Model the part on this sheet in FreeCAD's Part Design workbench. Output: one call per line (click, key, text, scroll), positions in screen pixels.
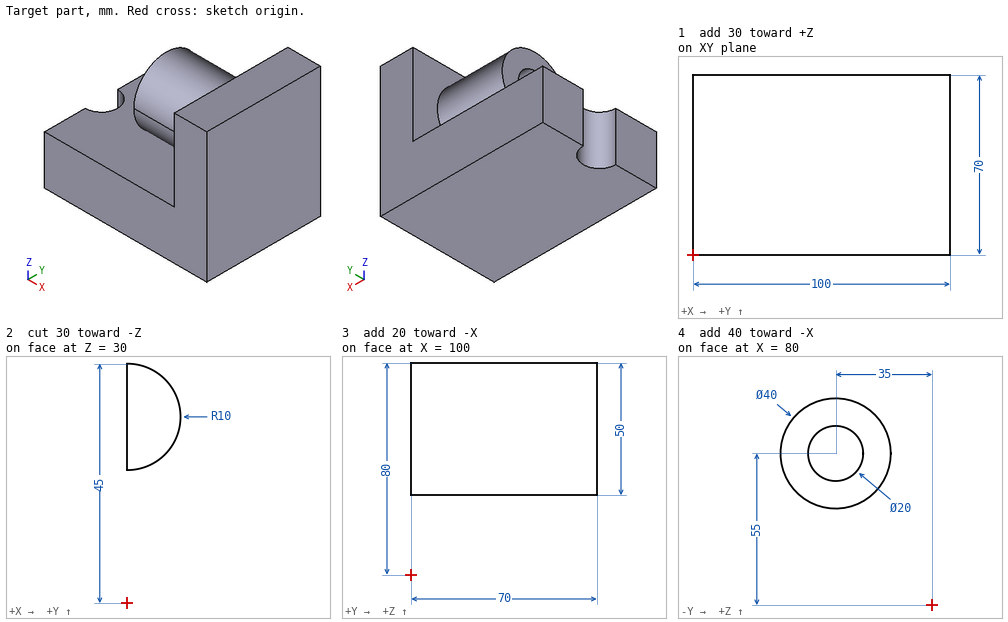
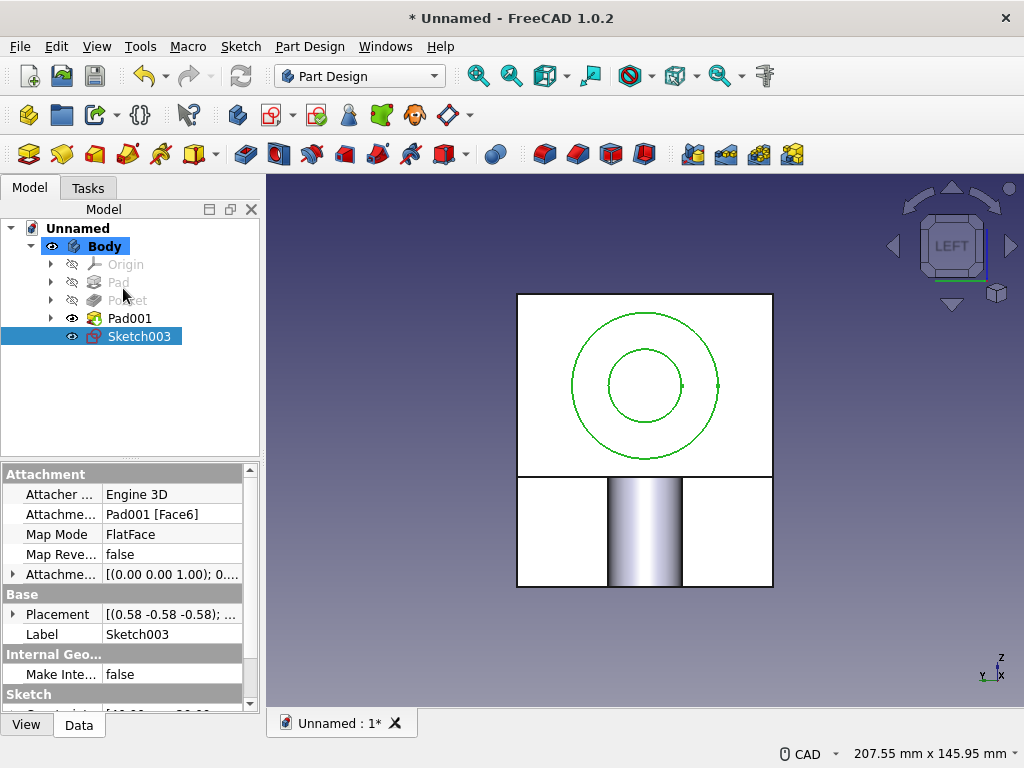
click(29, 154)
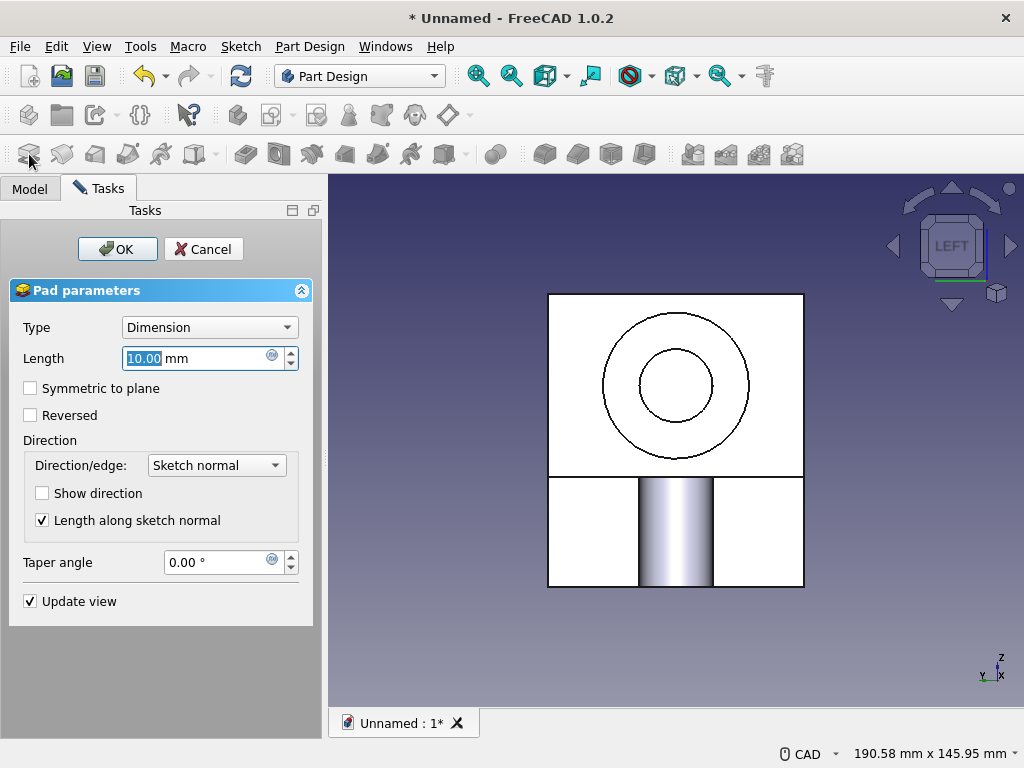
text(40)
key(Tab)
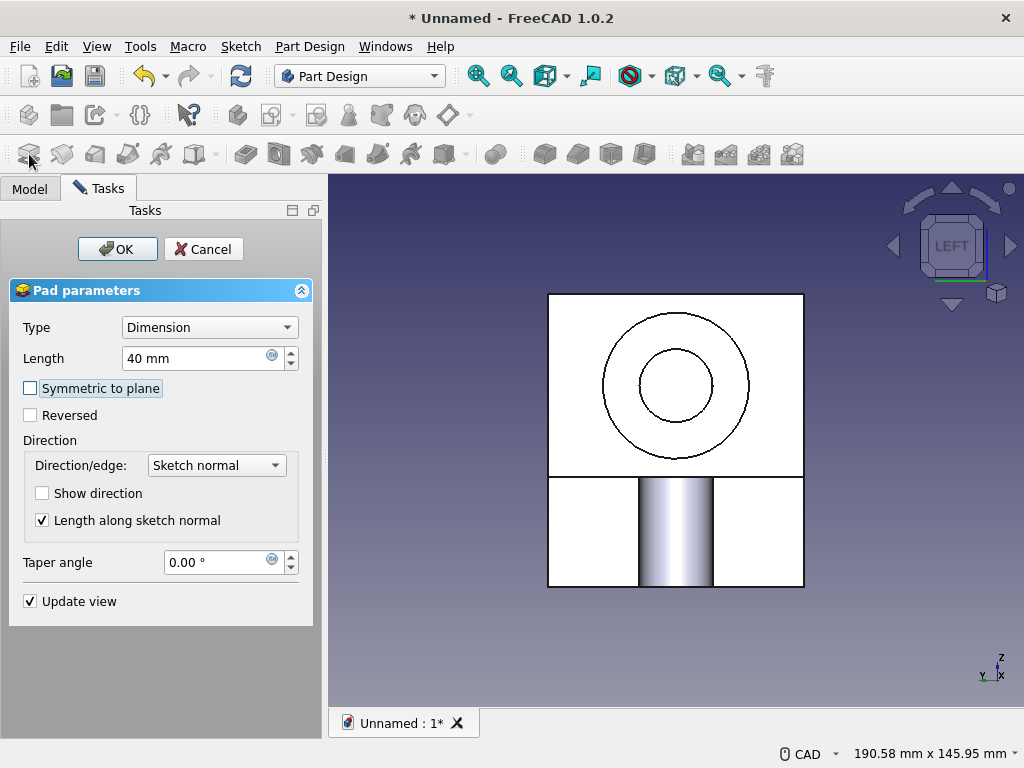
click(118, 249)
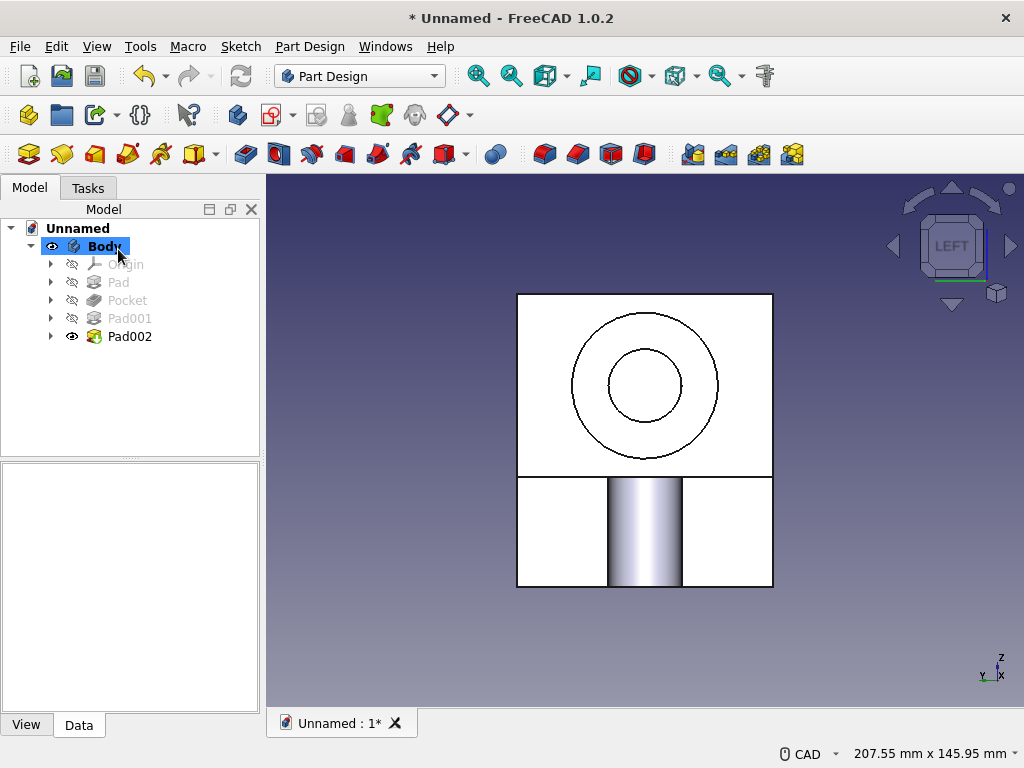
key(0)